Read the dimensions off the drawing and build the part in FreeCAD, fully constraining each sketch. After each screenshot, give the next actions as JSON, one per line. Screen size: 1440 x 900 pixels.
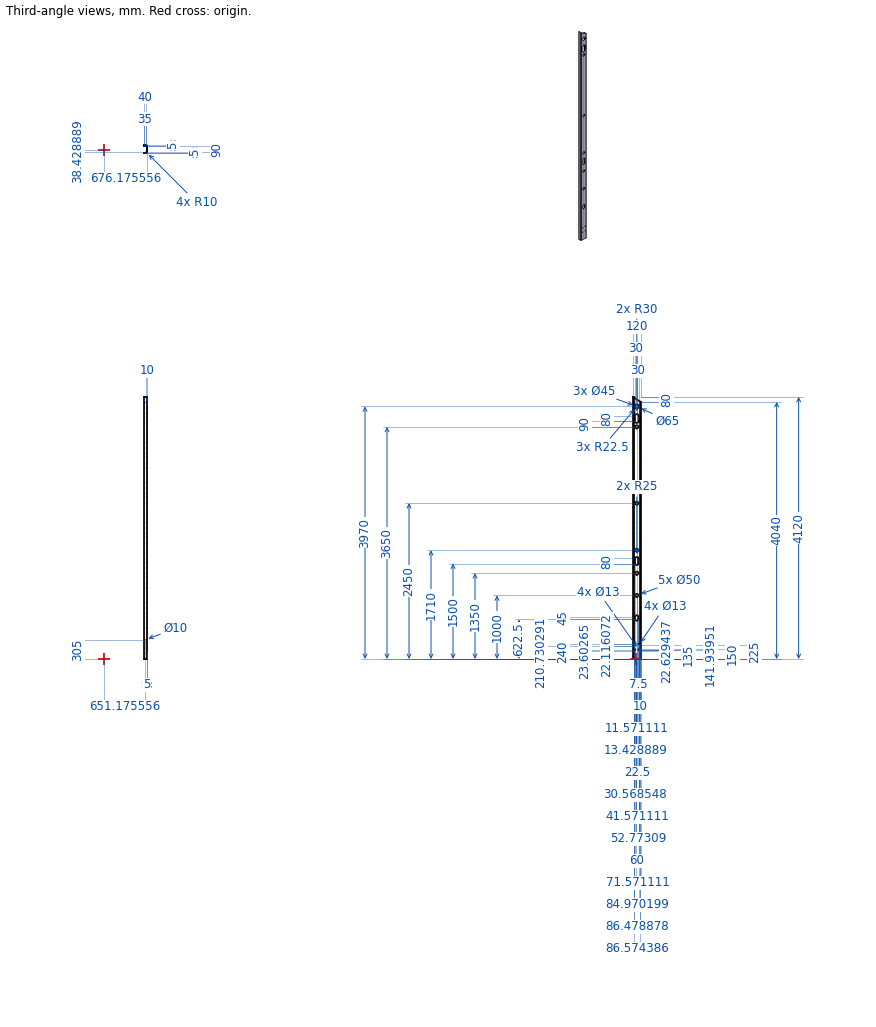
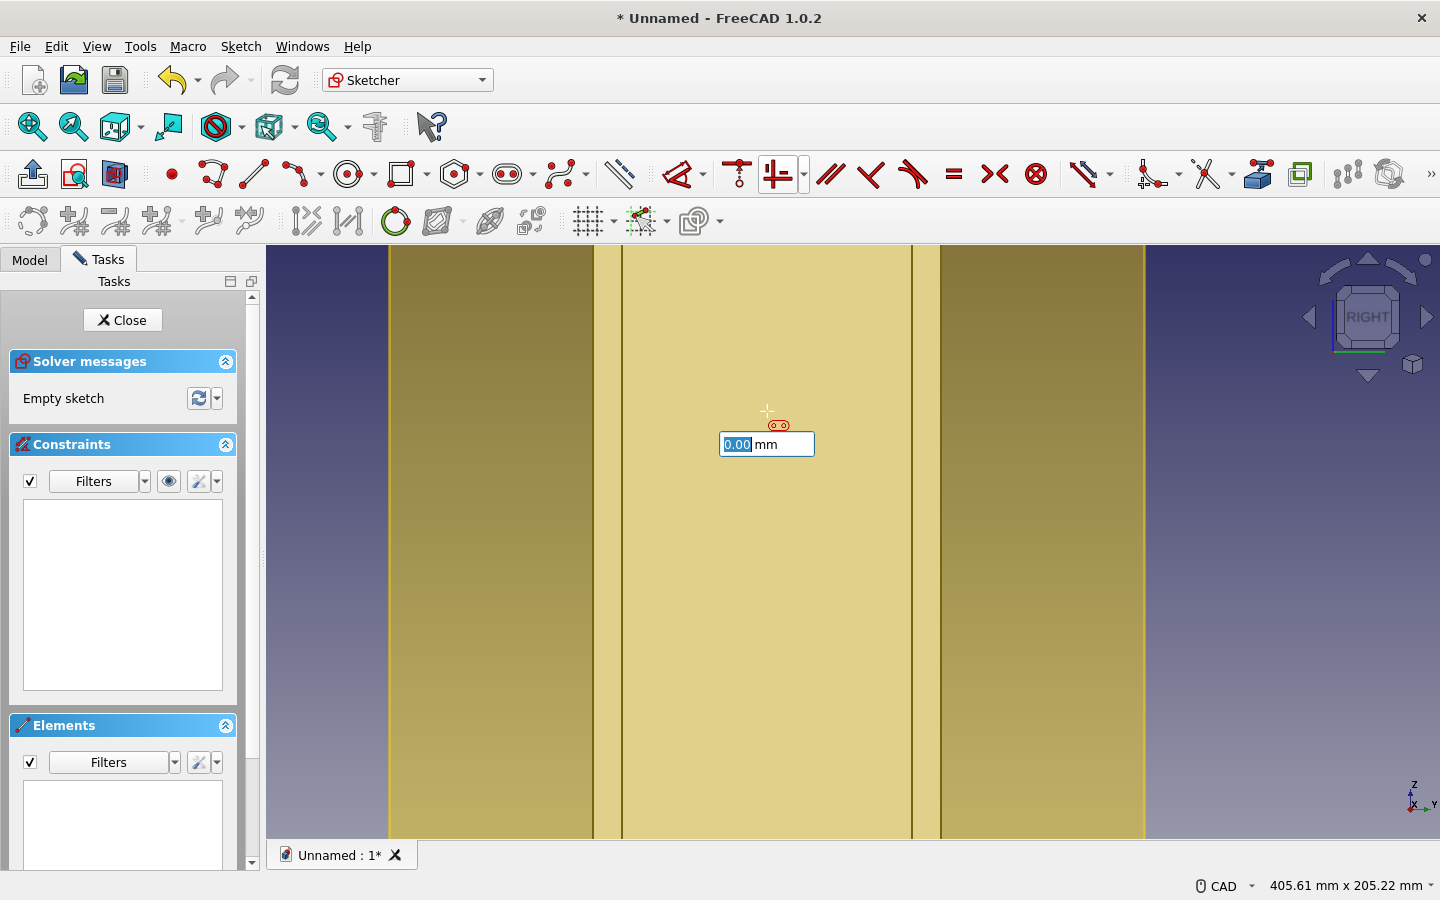
{"action": "left_click", "coordinate": [839, 527]}
{"action": "key", "text": "Escape"}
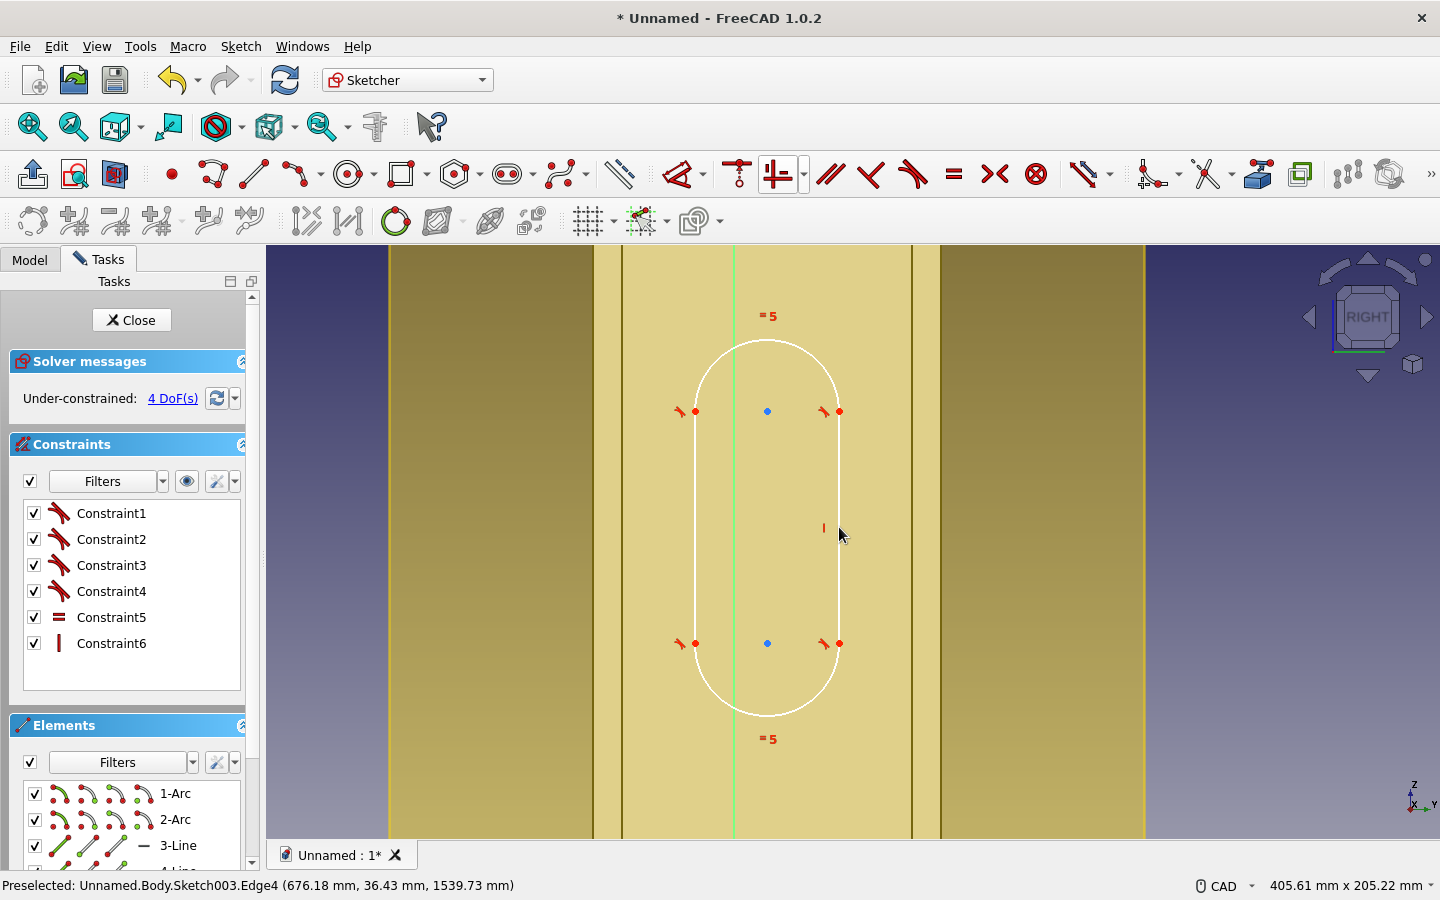
{"action": "left_click", "coordinate": [676, 174]}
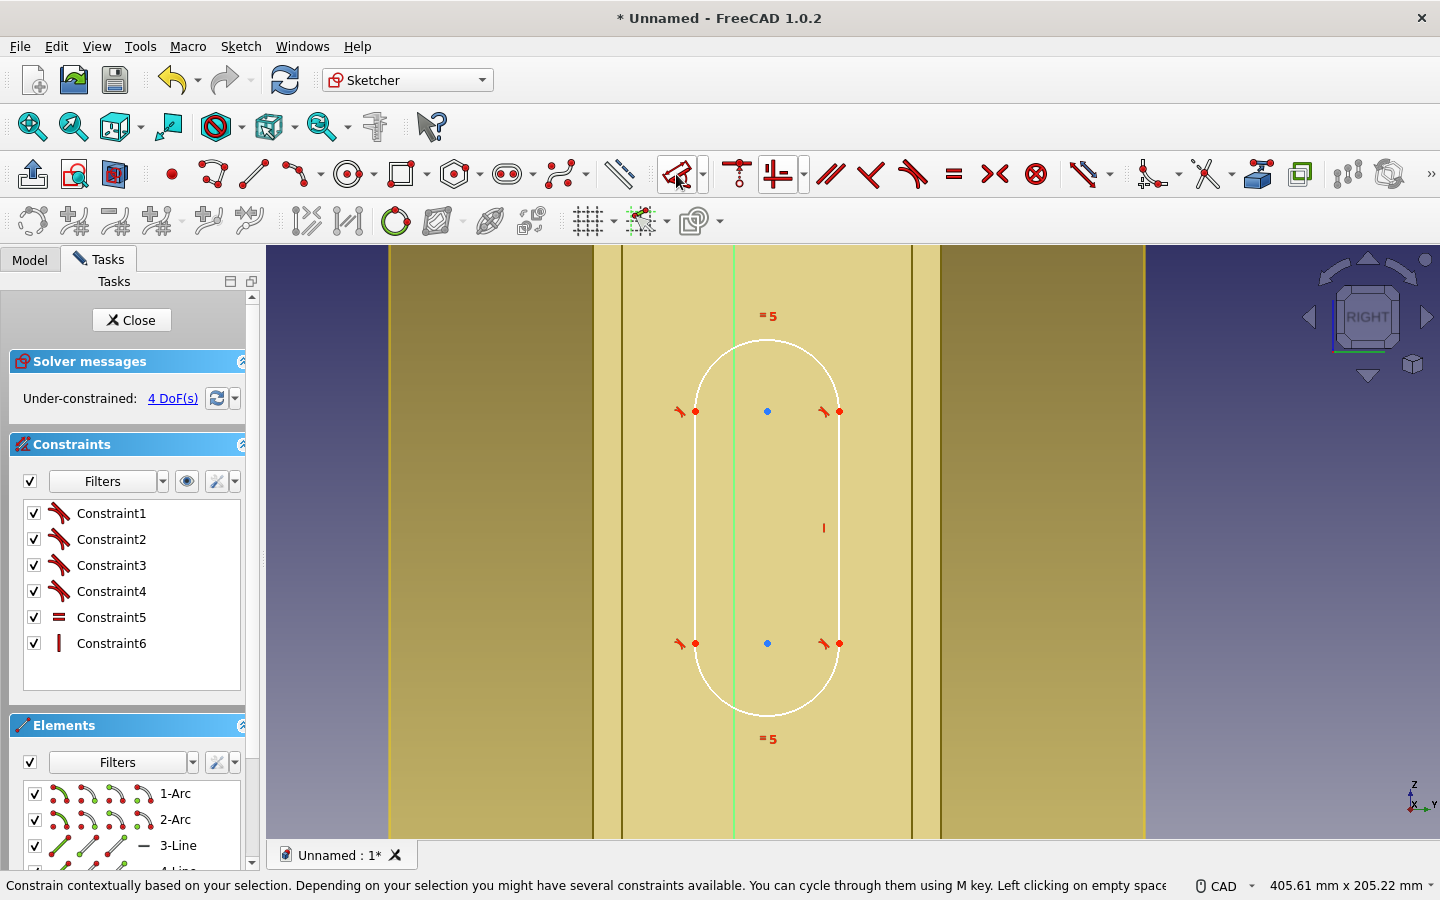
{"action": "left_click", "coordinate": [809, 702]}
{"action": "left_click", "coordinate": [828, 728]}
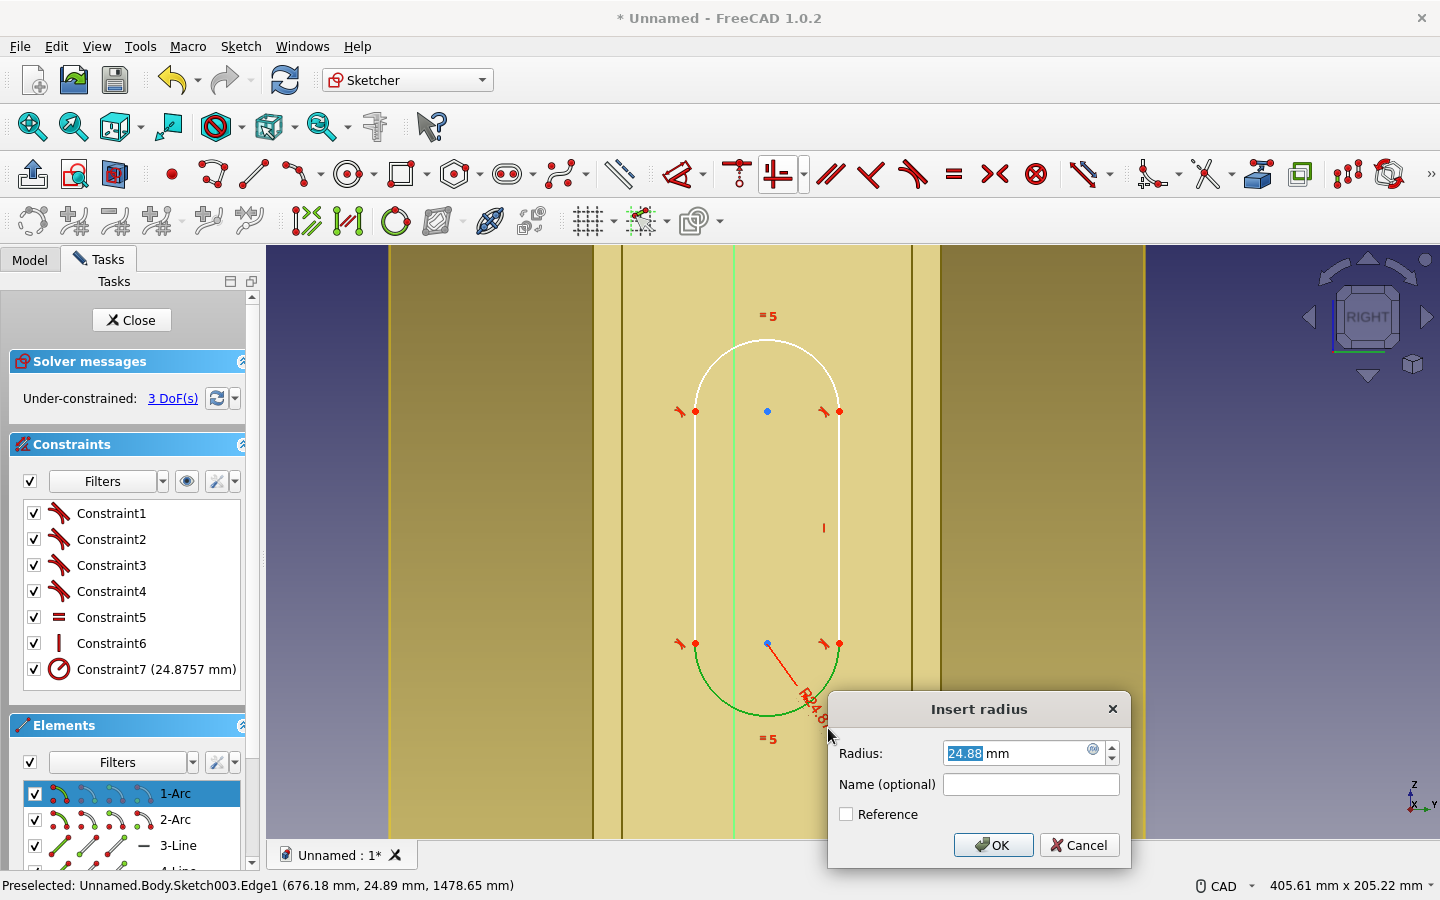
{"action": "type", "text": "25"}
{"action": "key", "text": "Return"}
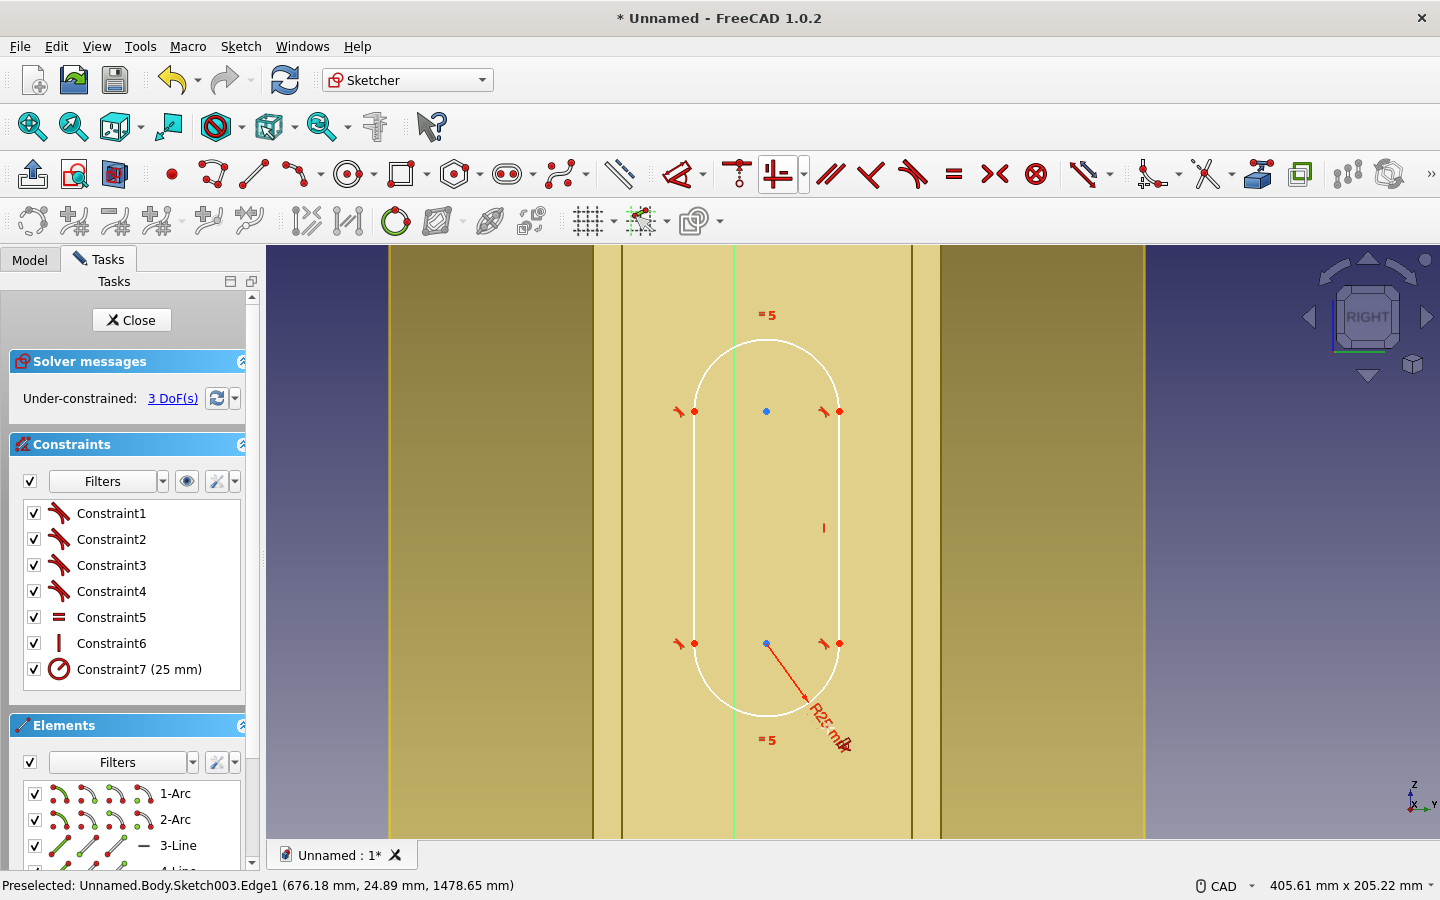
{"action": "left_click", "coordinate": [694, 574]}
{"action": "left_click", "coordinate": [660, 528]}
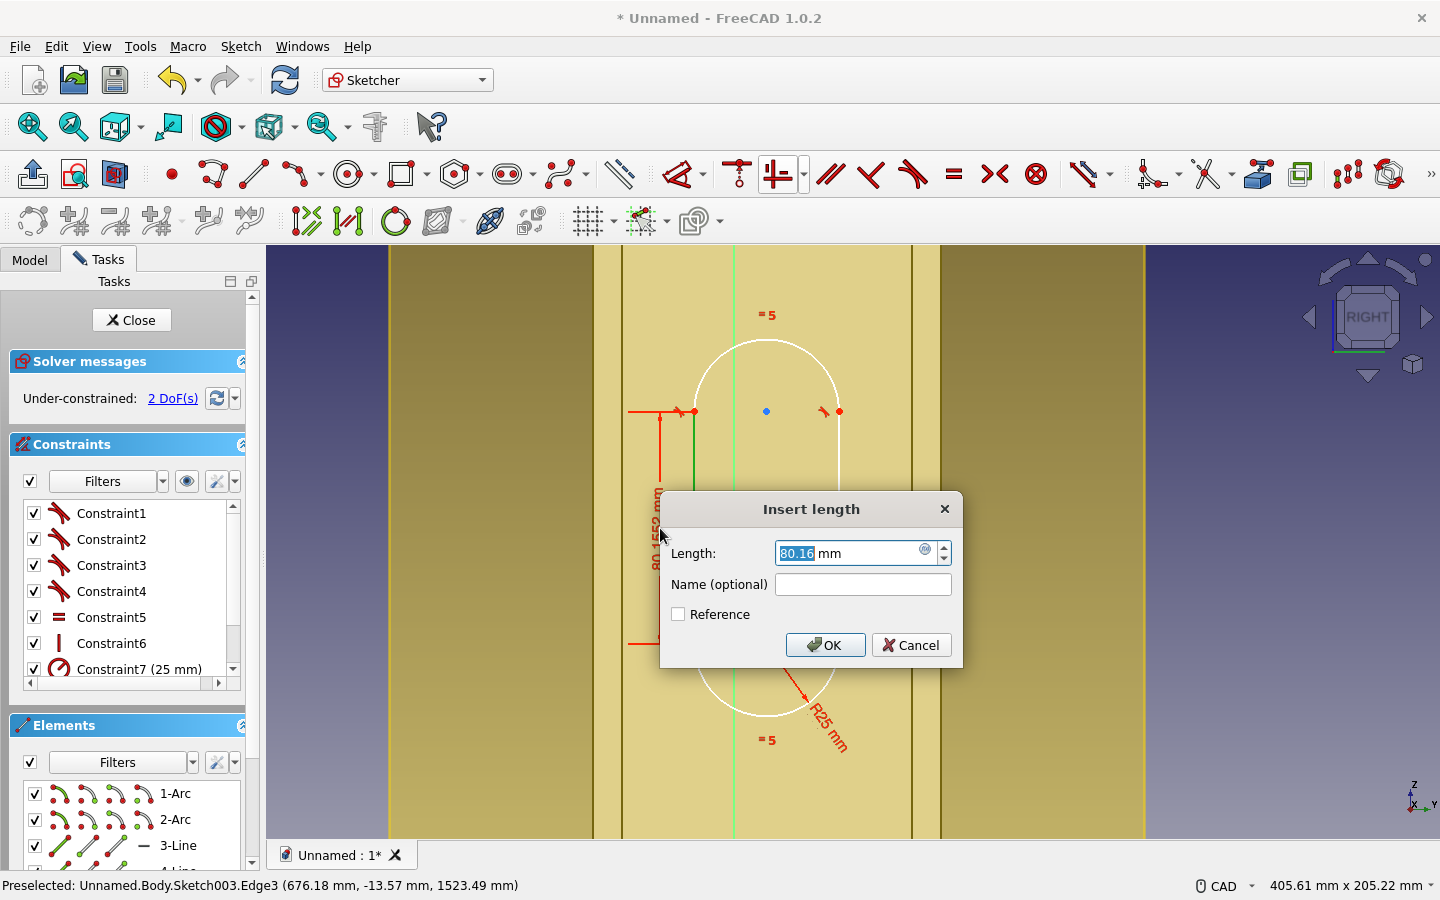
{"action": "type", "text": "80"}
{"action": "key", "text": "Return"}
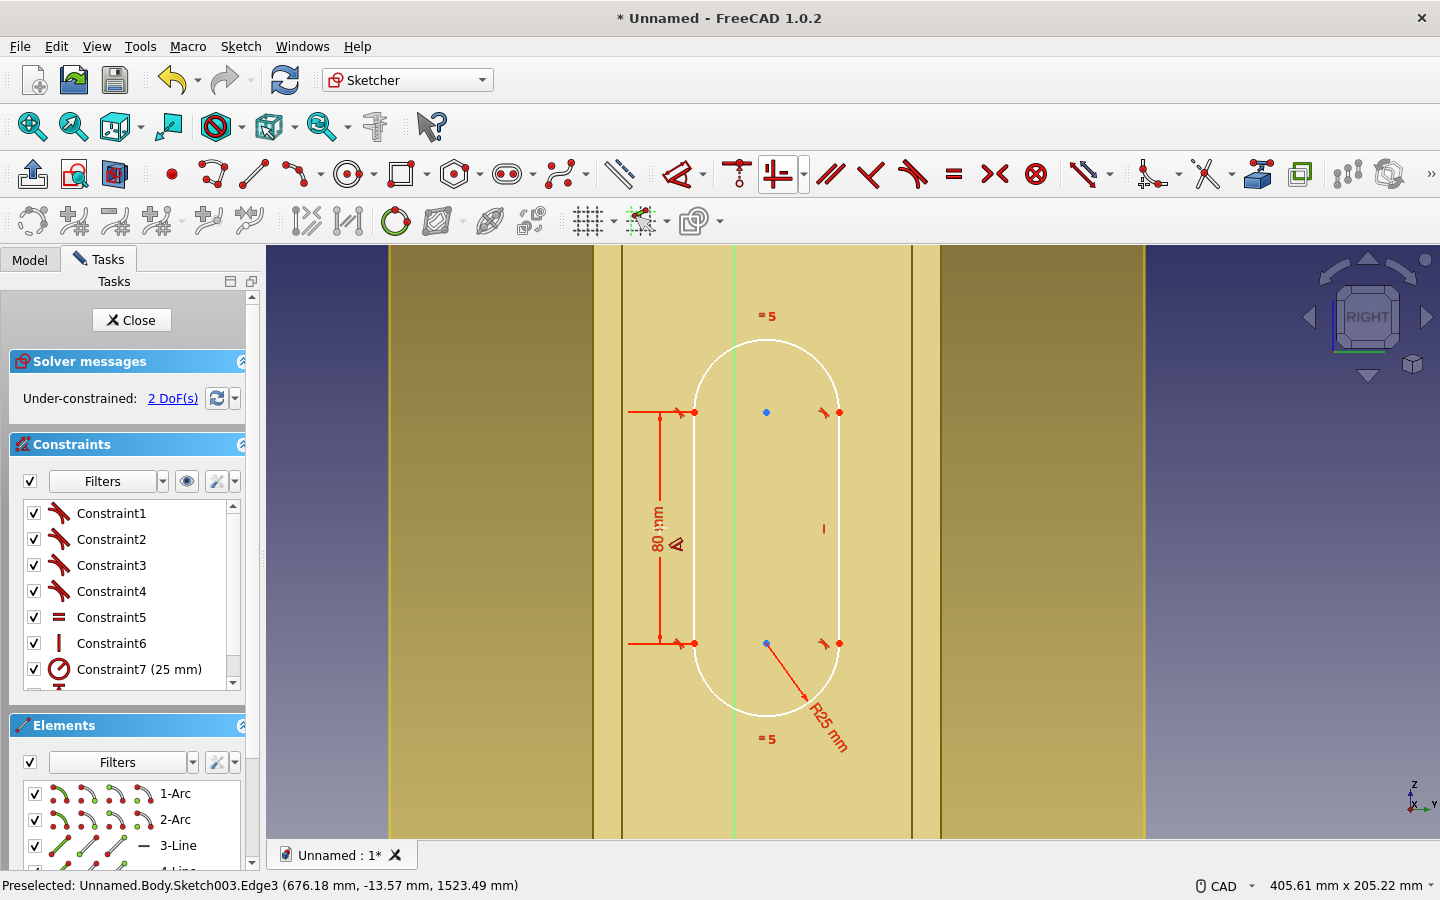
{"action": "left_click", "coordinate": [694, 644]}
{"action": "left_click", "coordinate": [660, 727]}